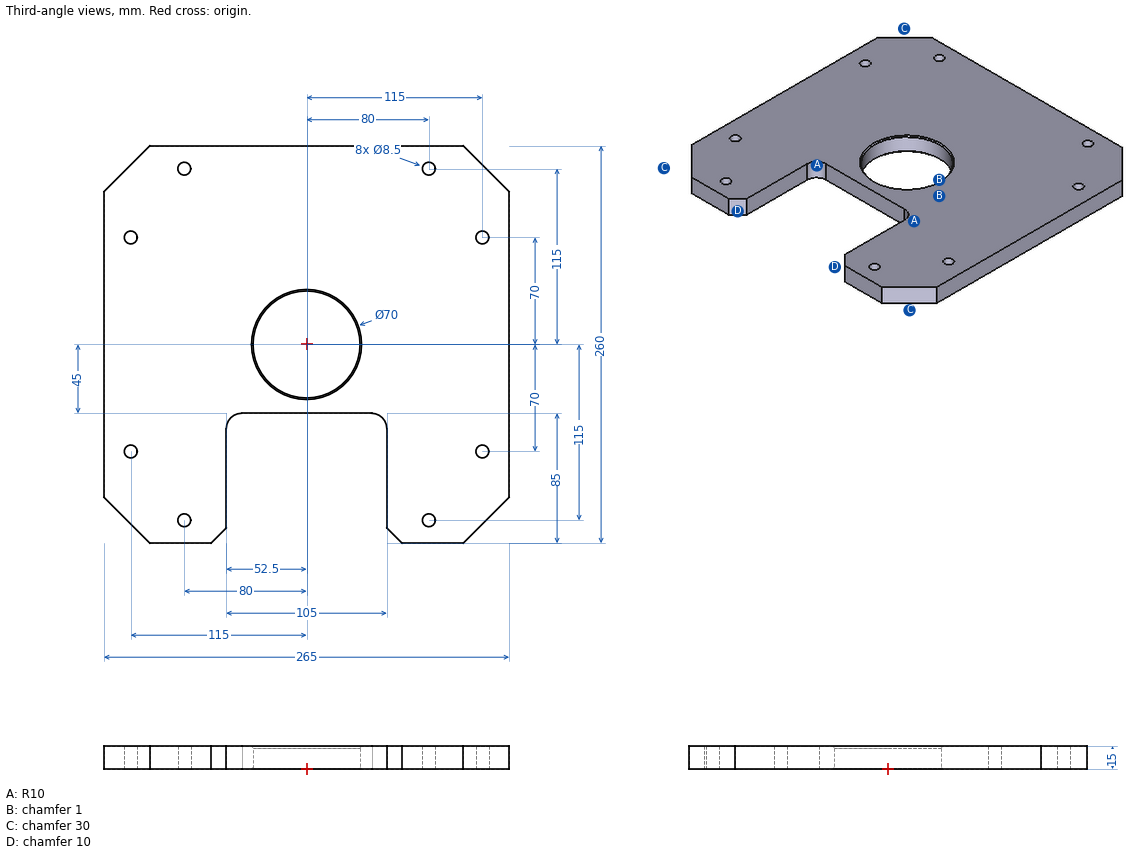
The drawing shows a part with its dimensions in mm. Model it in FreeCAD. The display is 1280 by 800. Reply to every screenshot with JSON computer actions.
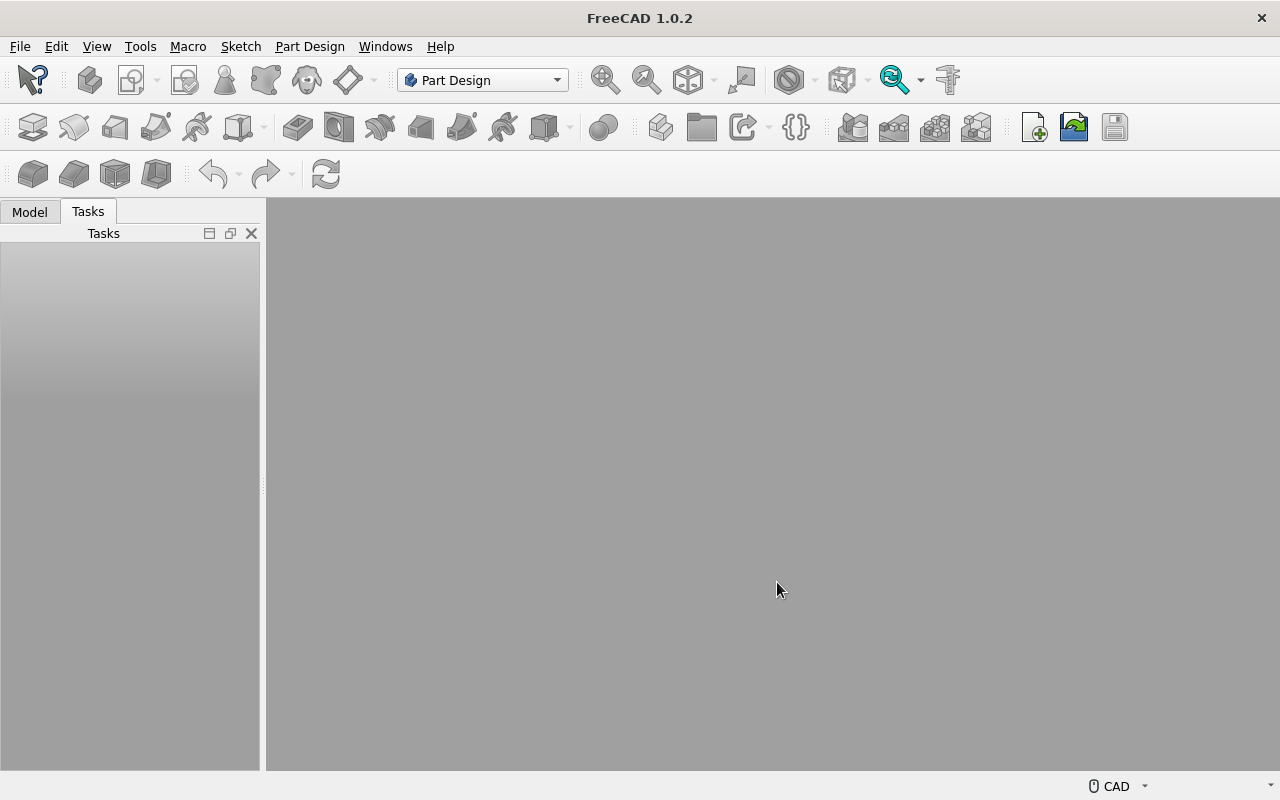
{"action": "left_click", "coordinate": [1033, 128]}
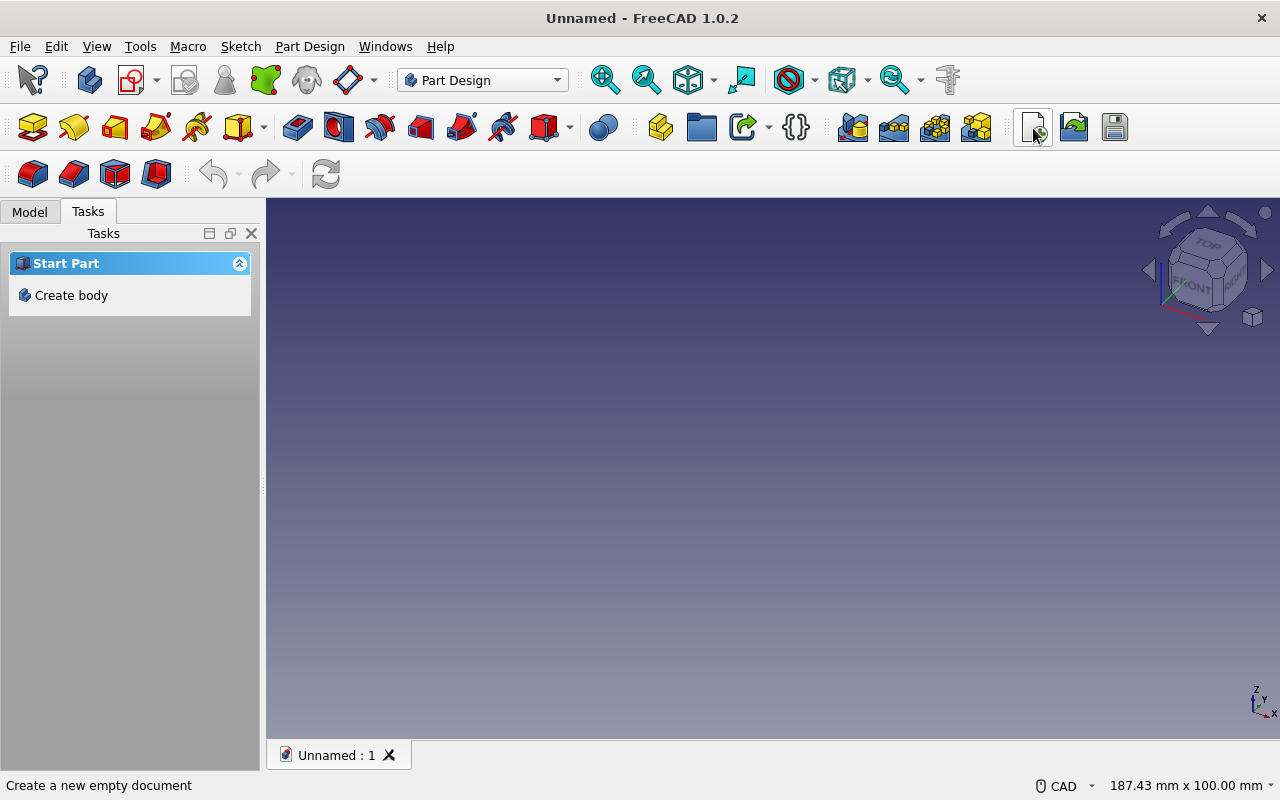
{"action": "left_click", "coordinate": [130, 80]}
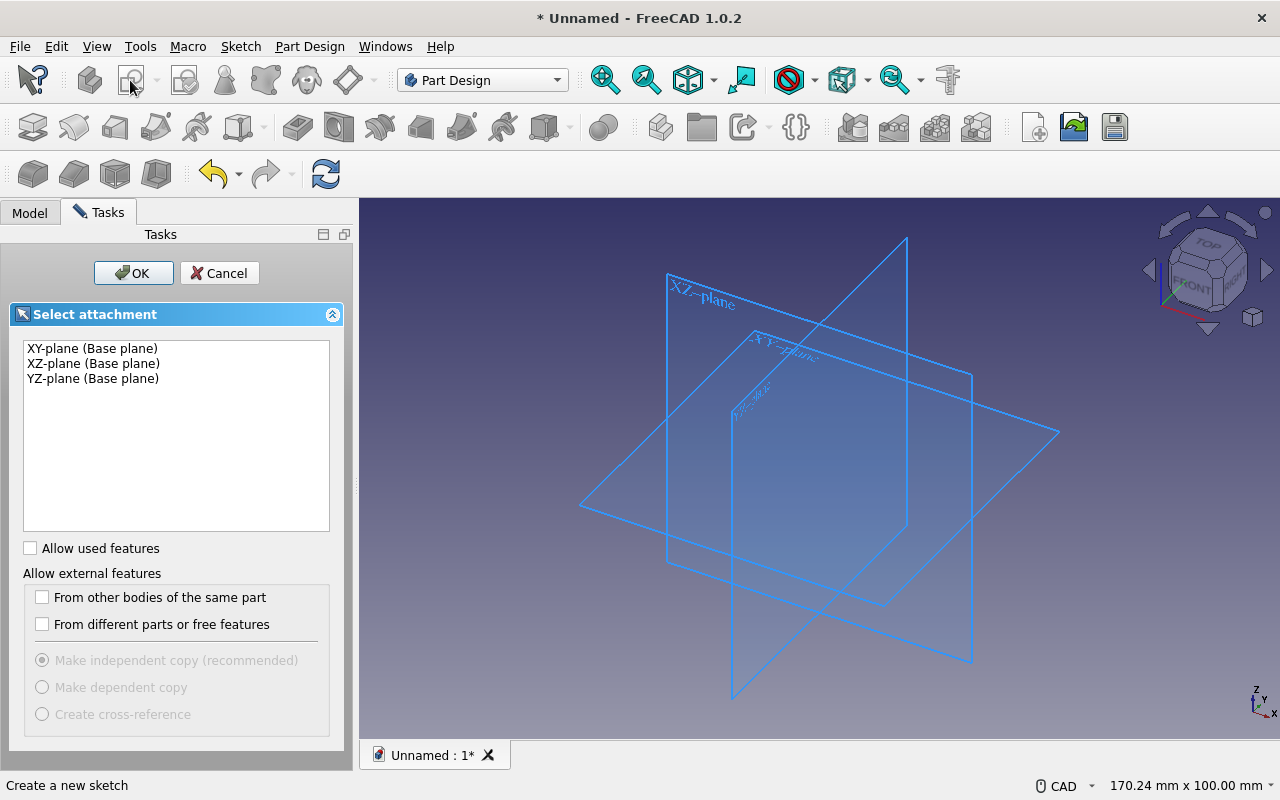
{"action": "left_click", "coordinate": [84, 348]}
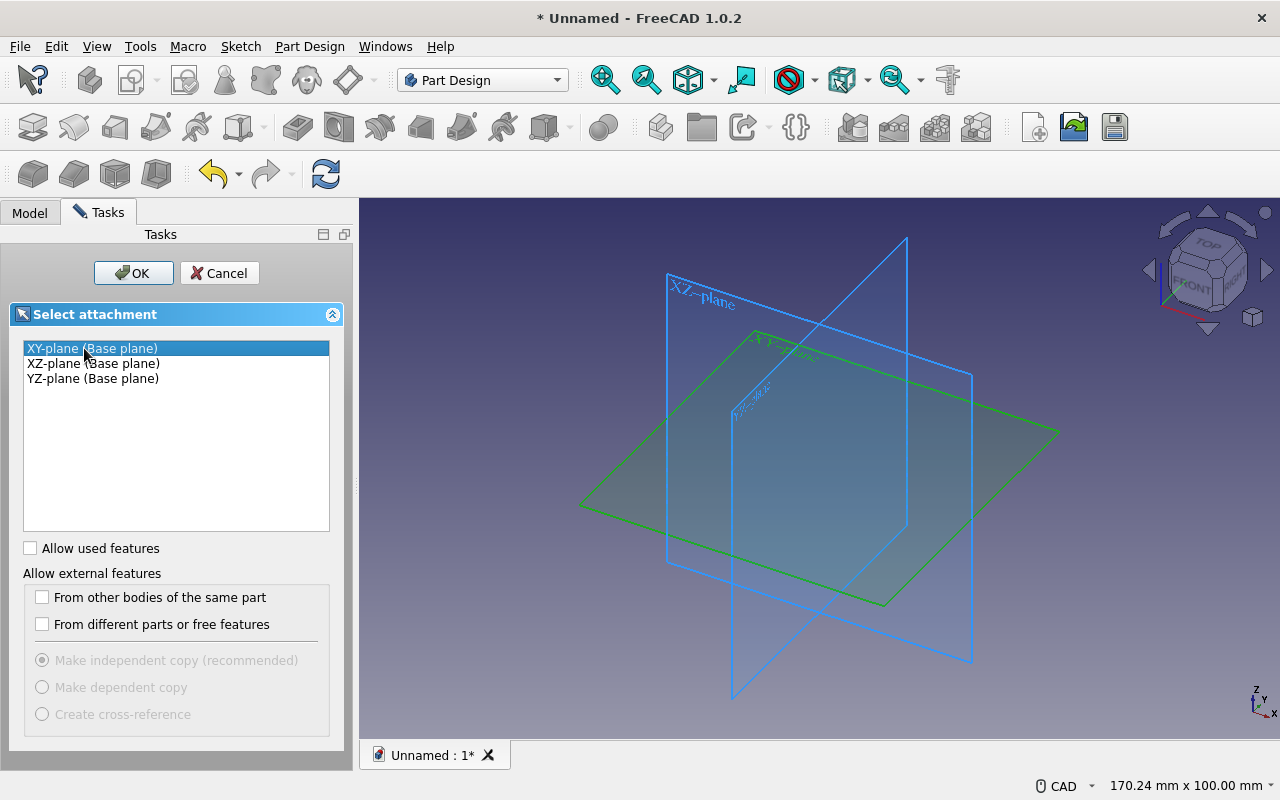
{"action": "left_click", "coordinate": [134, 273]}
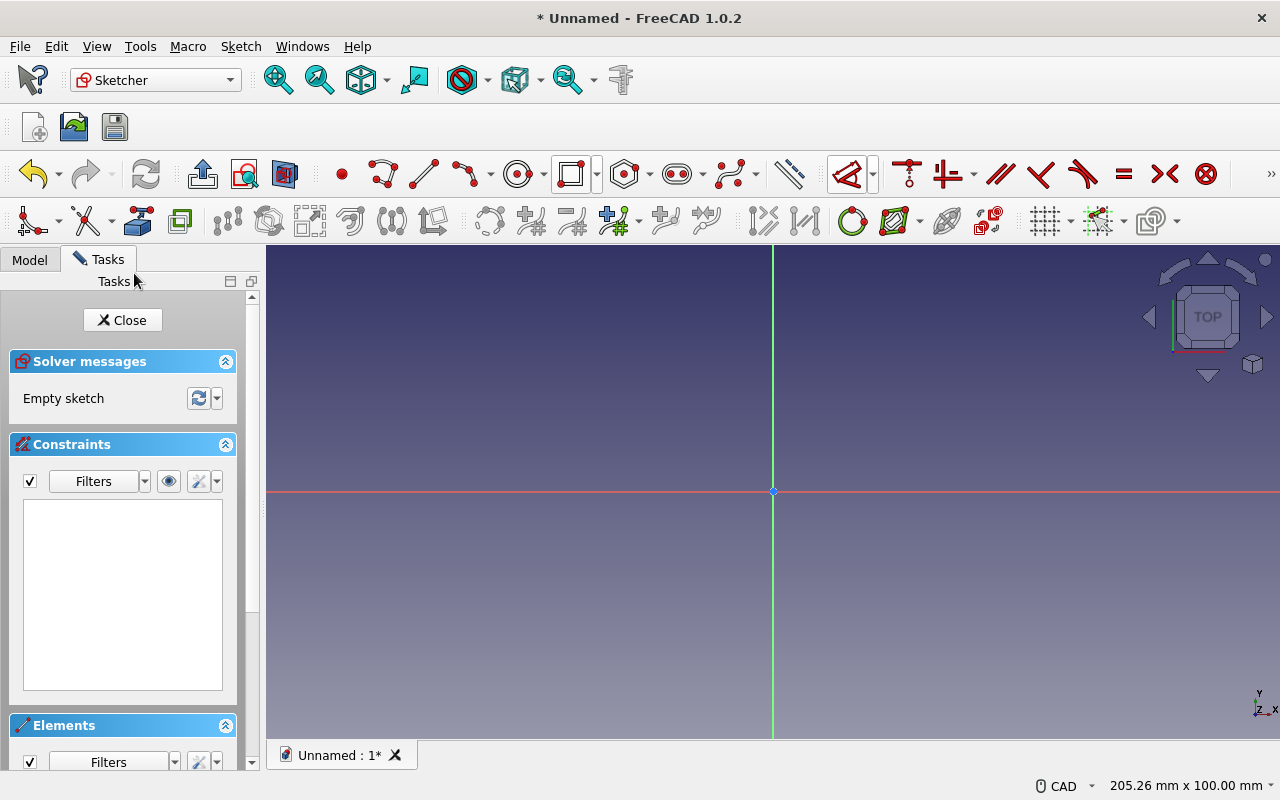
{"action": "scroll", "coordinate": [682, 492], "scroll_direction": "down", "scroll_amount": 7}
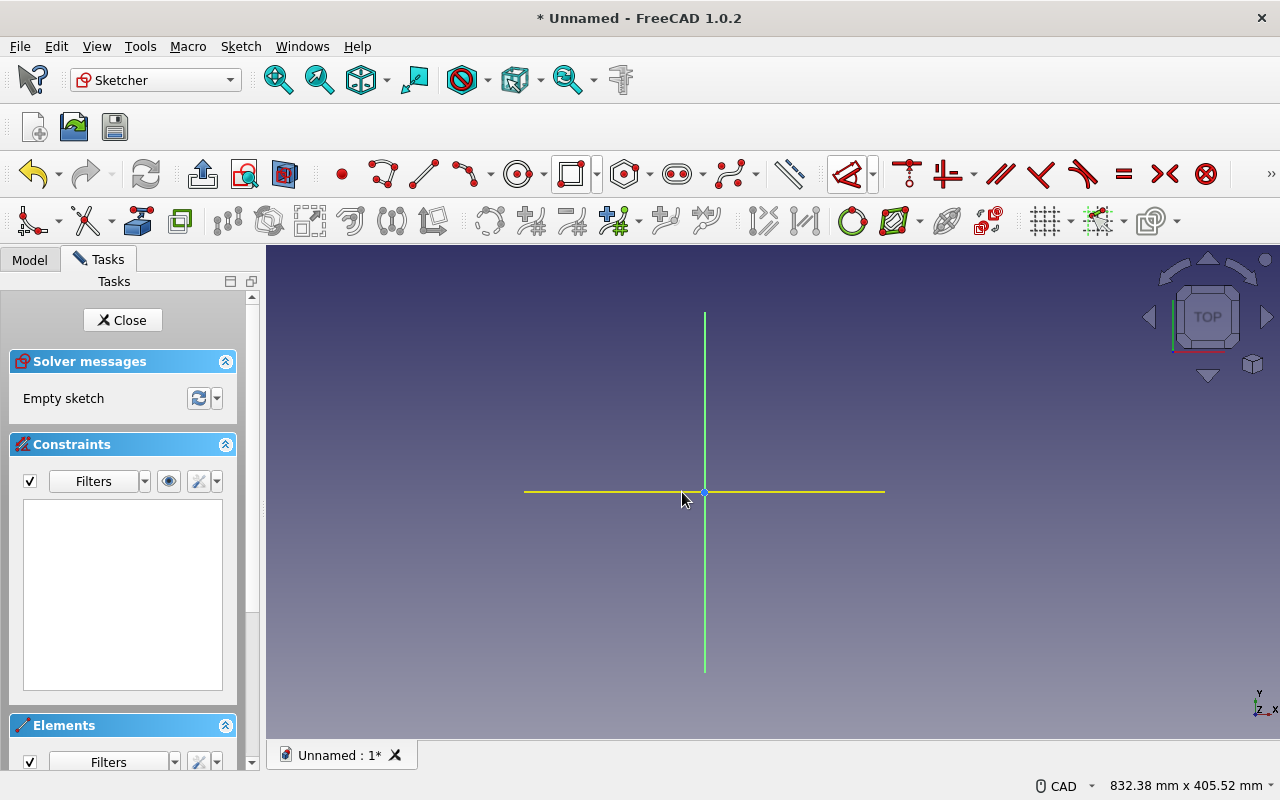
{"action": "key", "text": "g v"}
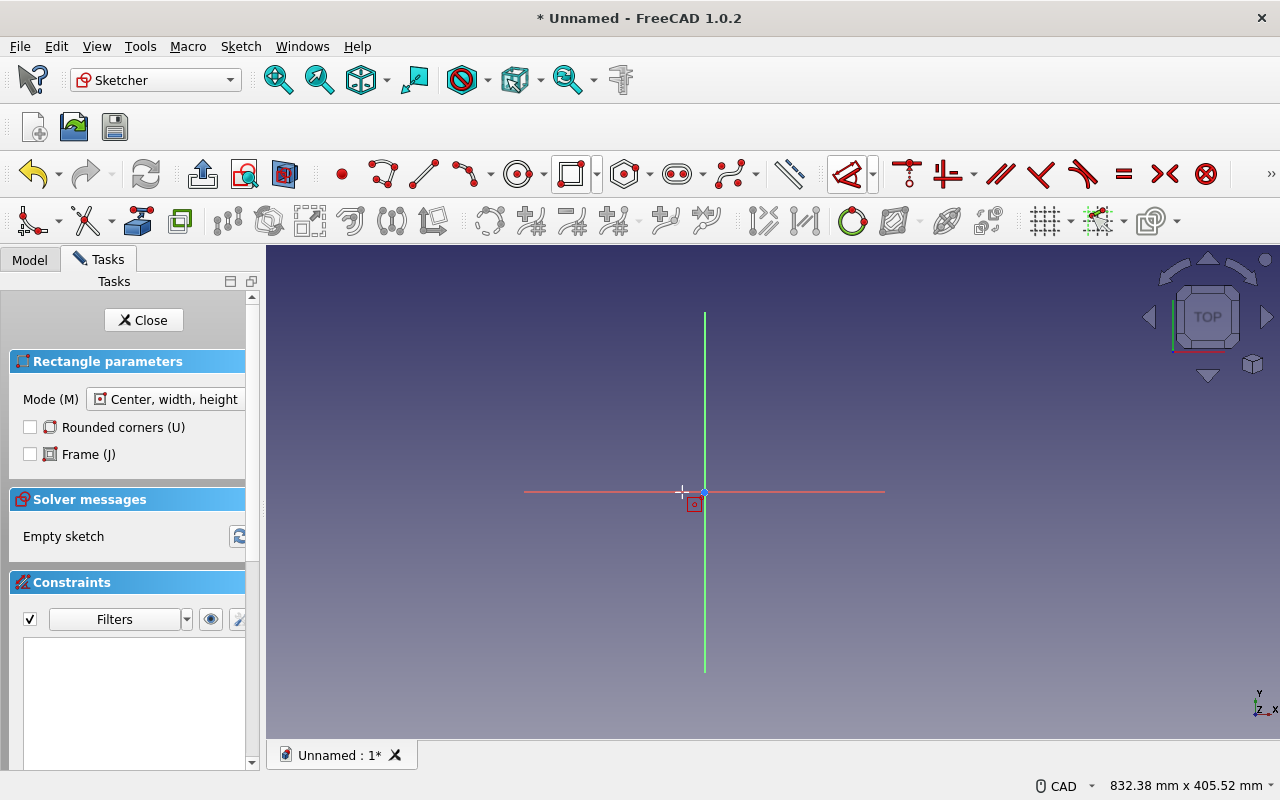
{"action": "left_click", "coordinate": [705, 492]}
{"action": "mouse_move", "coordinate": [866, 334]}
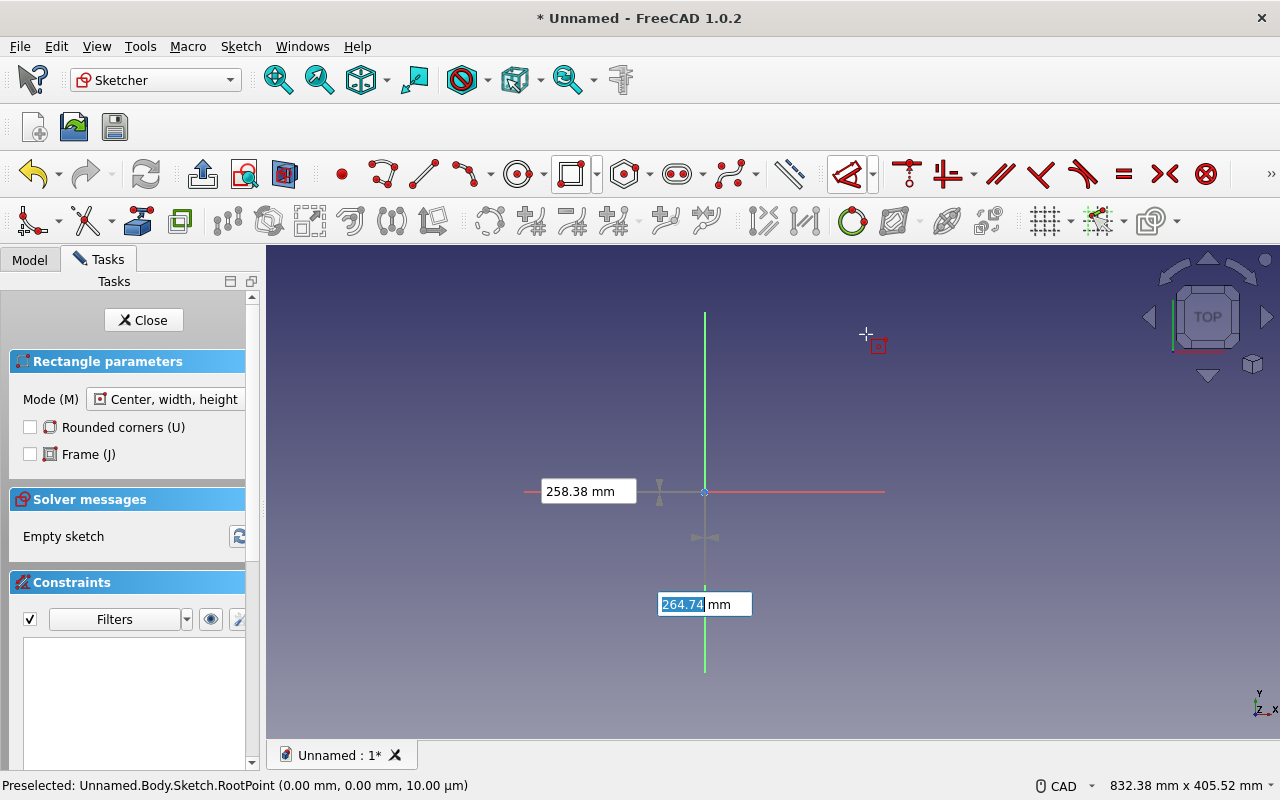
{"action": "type", "text": "265"}
{"action": "key", "text": "Tab"}
{"action": "type", "text": "260"}
{"action": "key", "text": "Return"}
{"action": "key", "text": "Escape"}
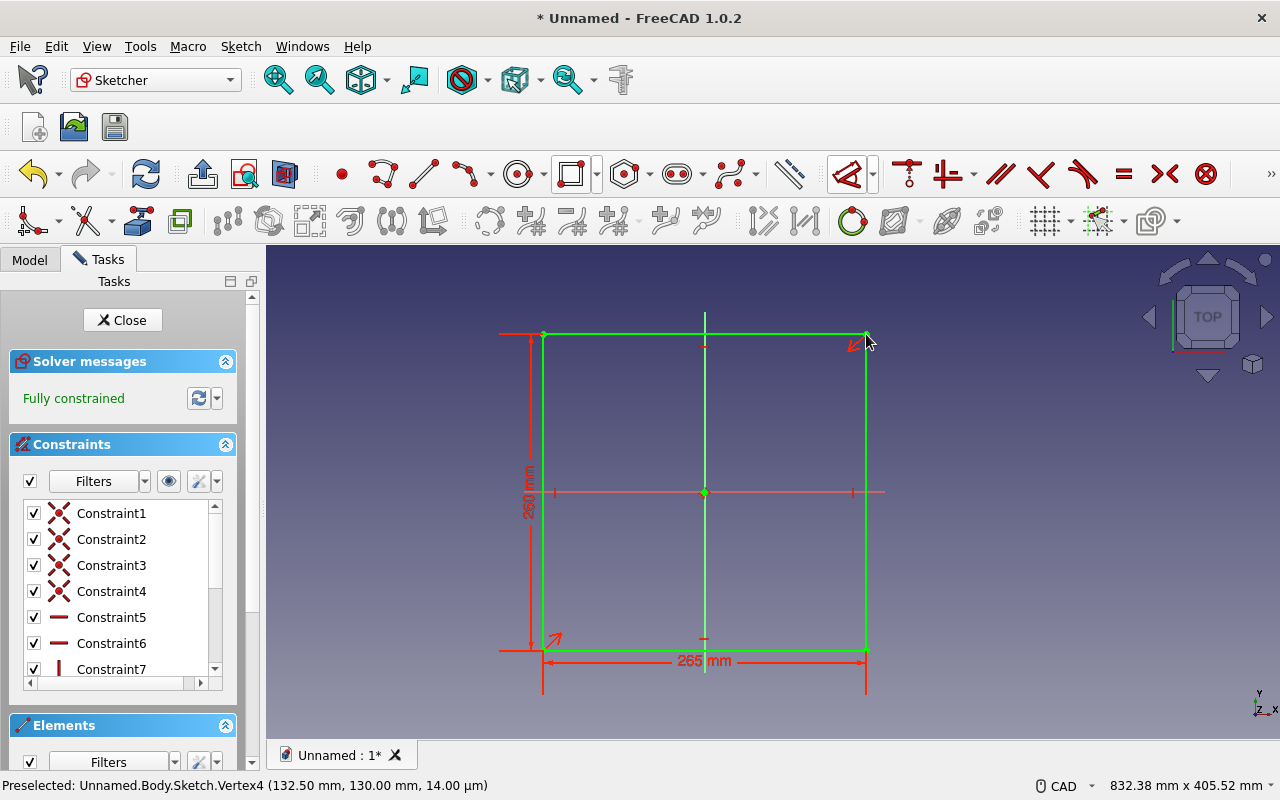
{"action": "left_click", "coordinate": [123, 320]}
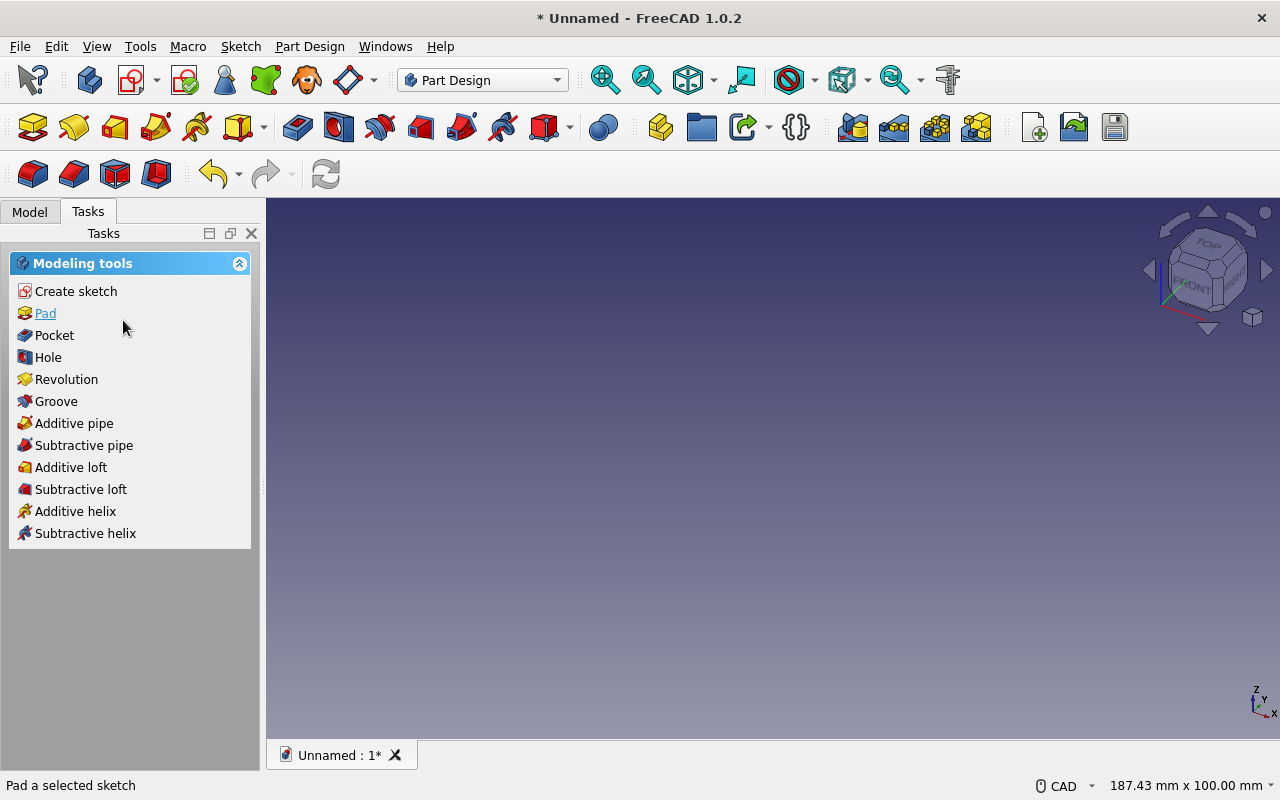
{"action": "left_click", "coordinate": [33, 128]}